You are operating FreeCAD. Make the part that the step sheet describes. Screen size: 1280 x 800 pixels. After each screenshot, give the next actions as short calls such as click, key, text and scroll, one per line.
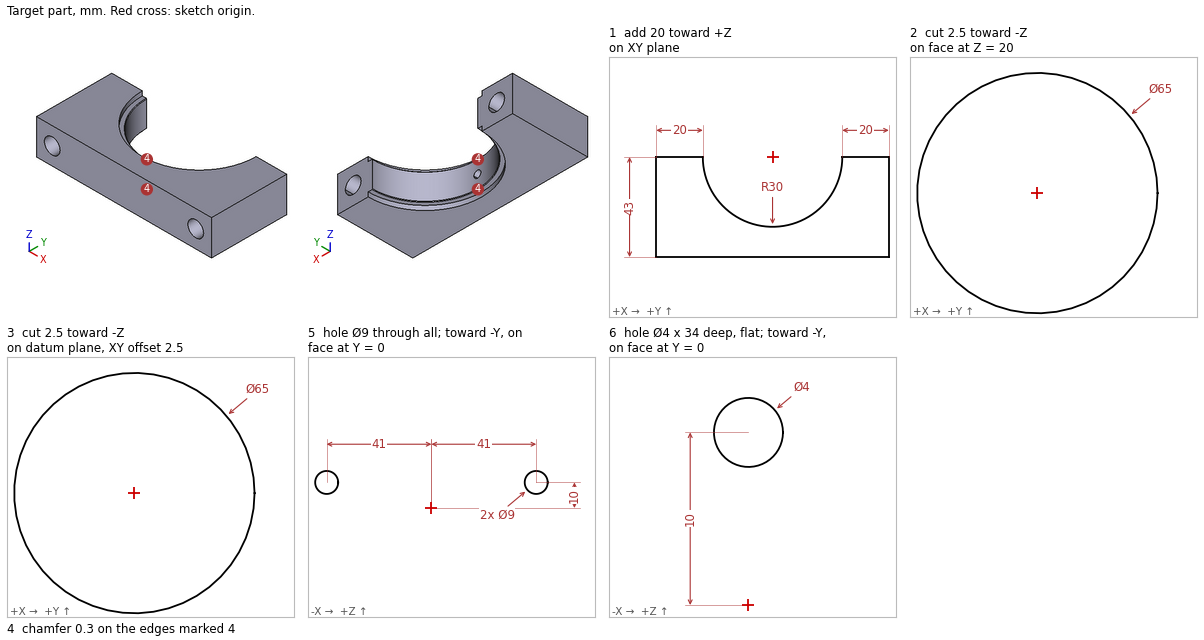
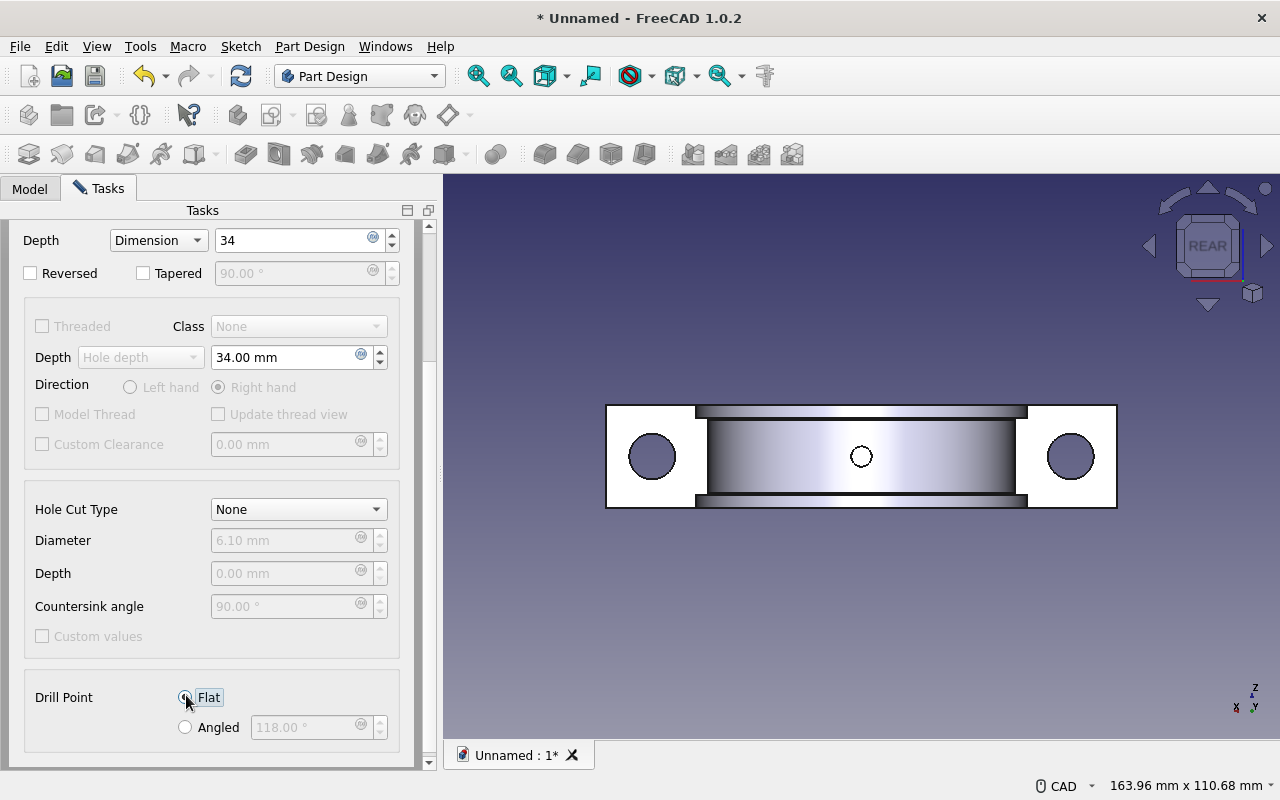
scroll(429, 495, up, 4)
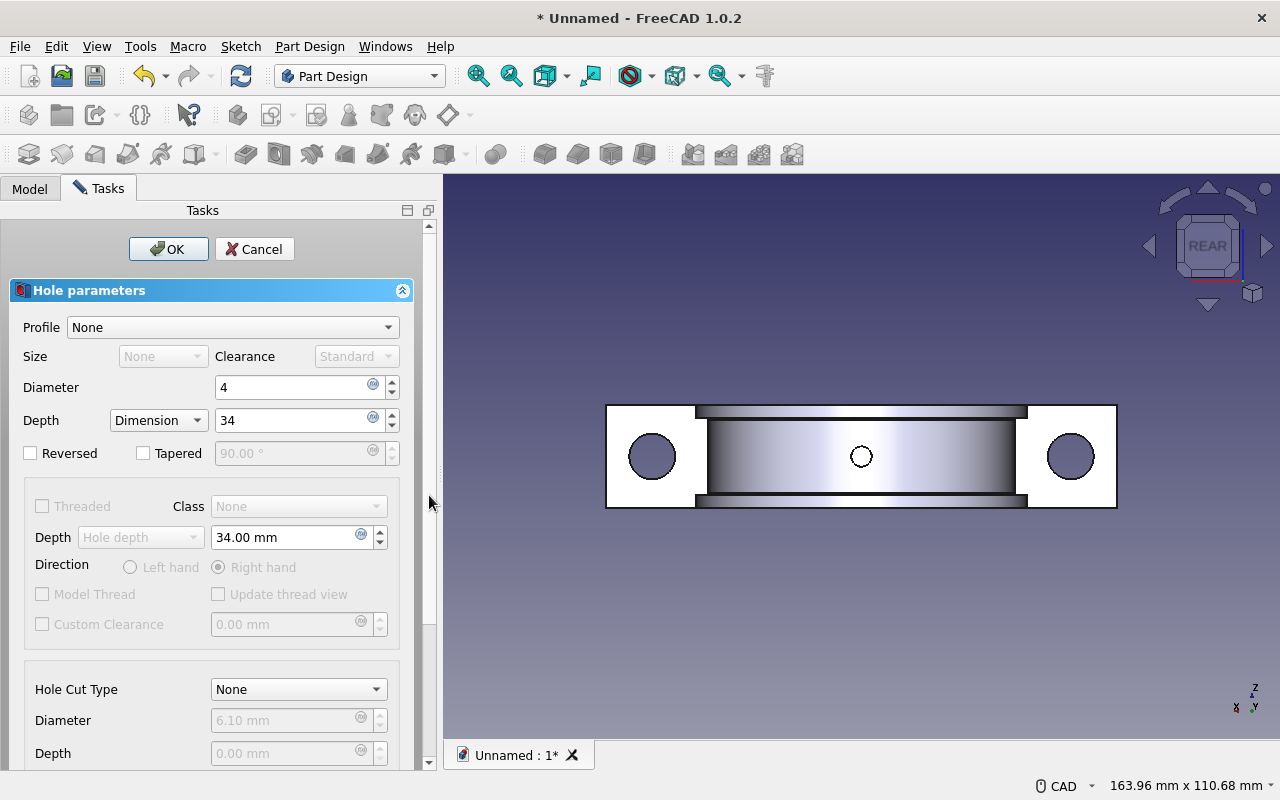
click(169, 249)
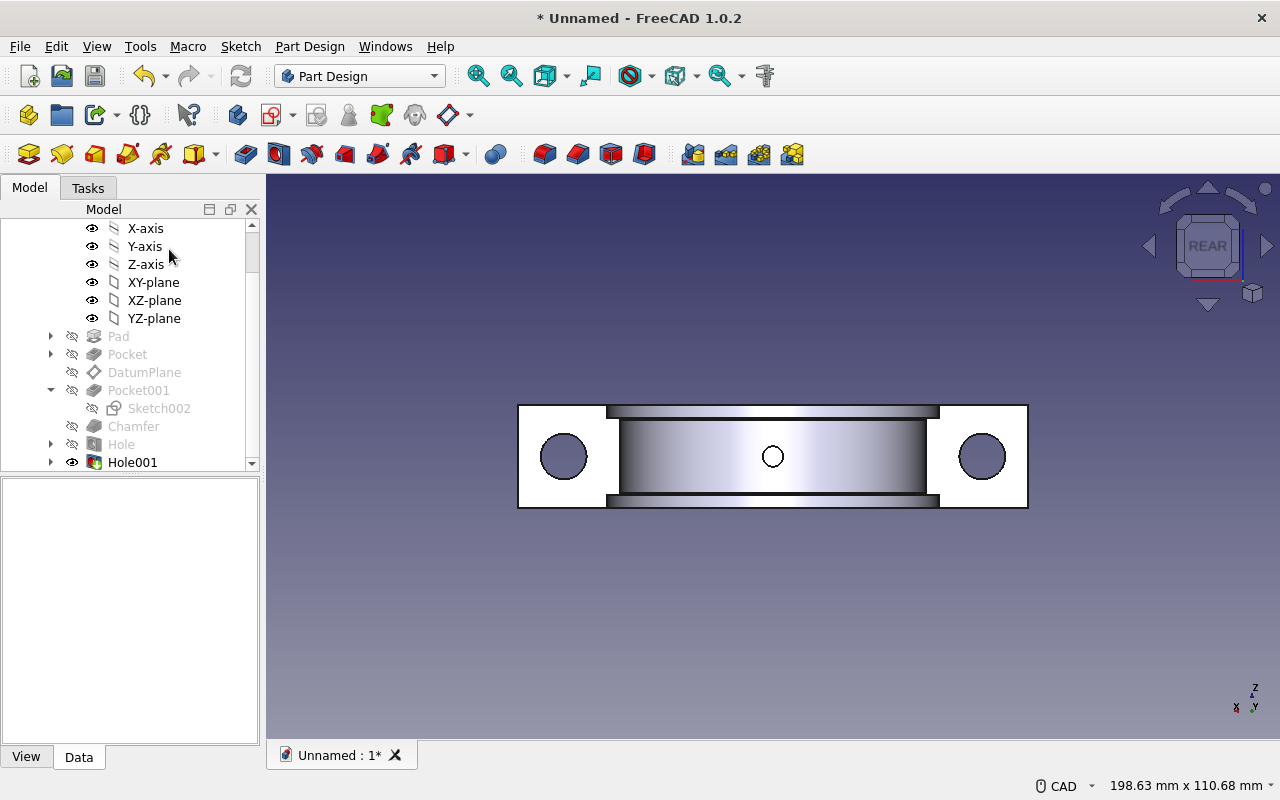
key(0)